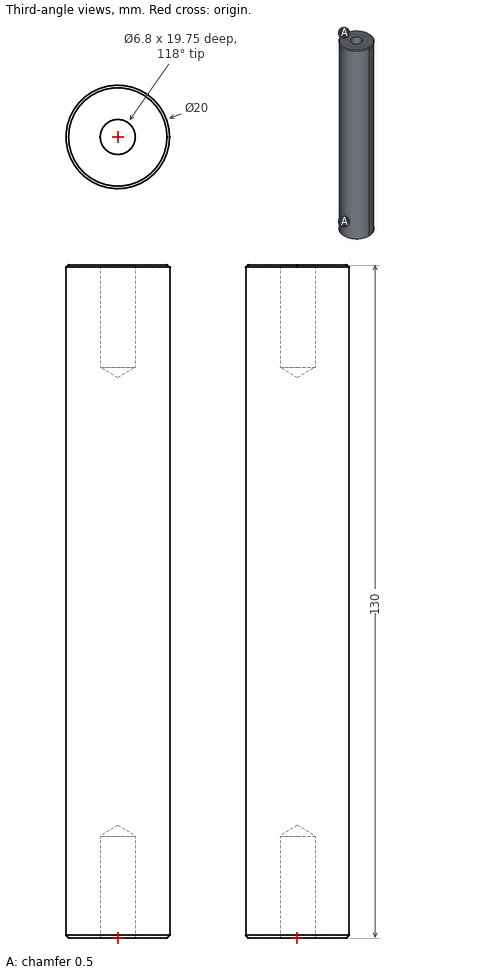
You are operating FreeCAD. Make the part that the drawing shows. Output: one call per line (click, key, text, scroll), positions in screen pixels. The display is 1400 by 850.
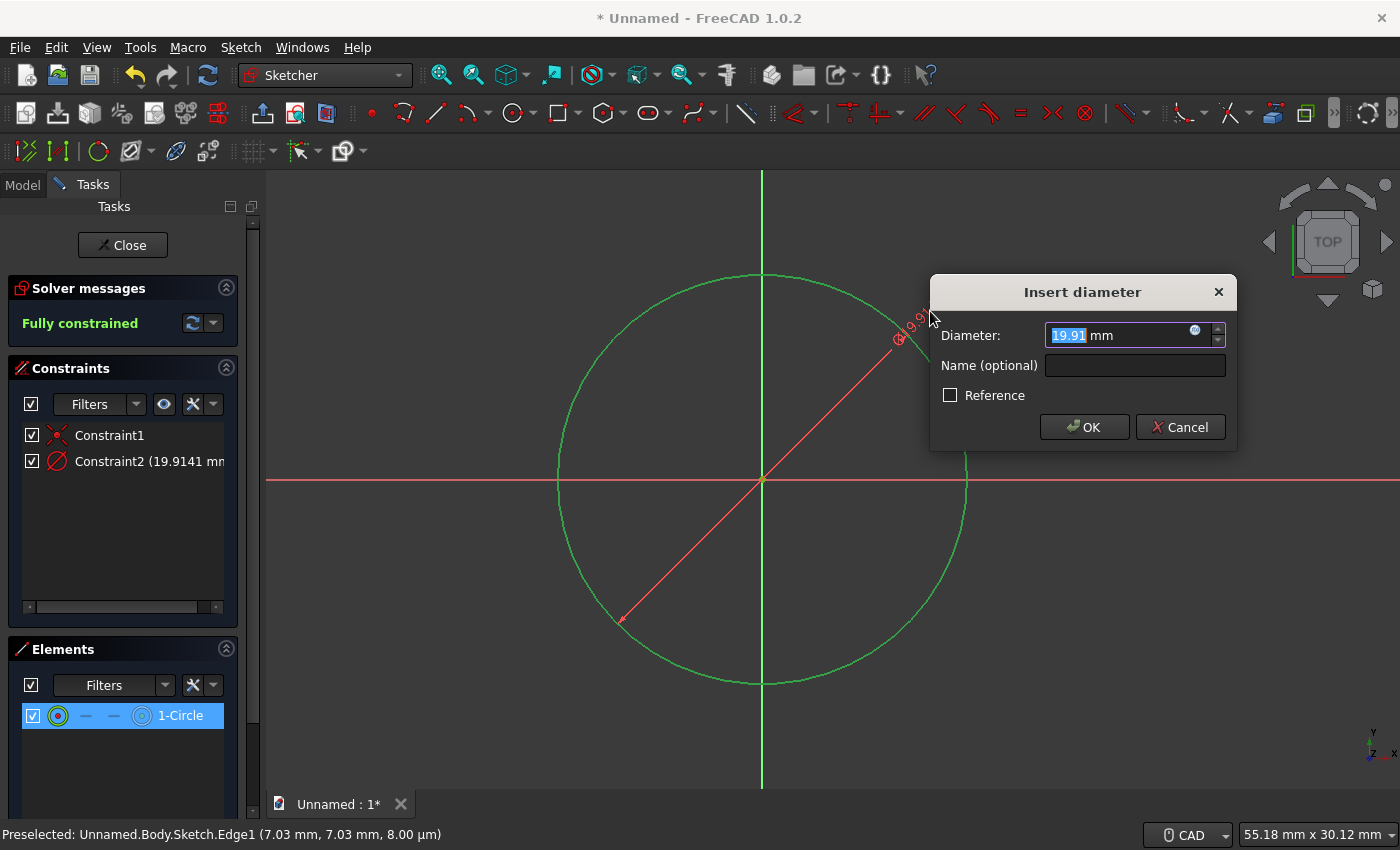
text(20)
key(Return)
key(Escape)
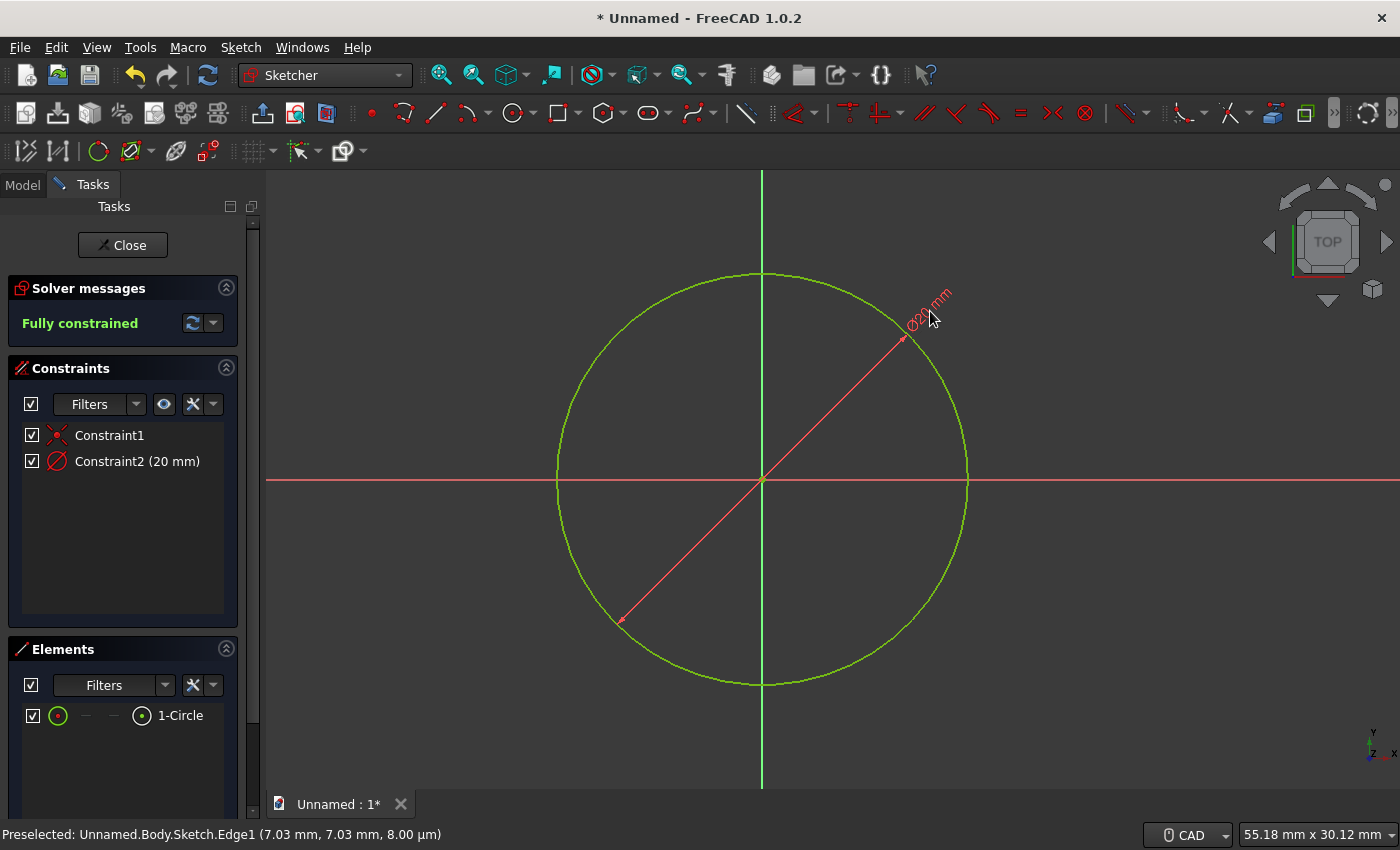
click(123, 245)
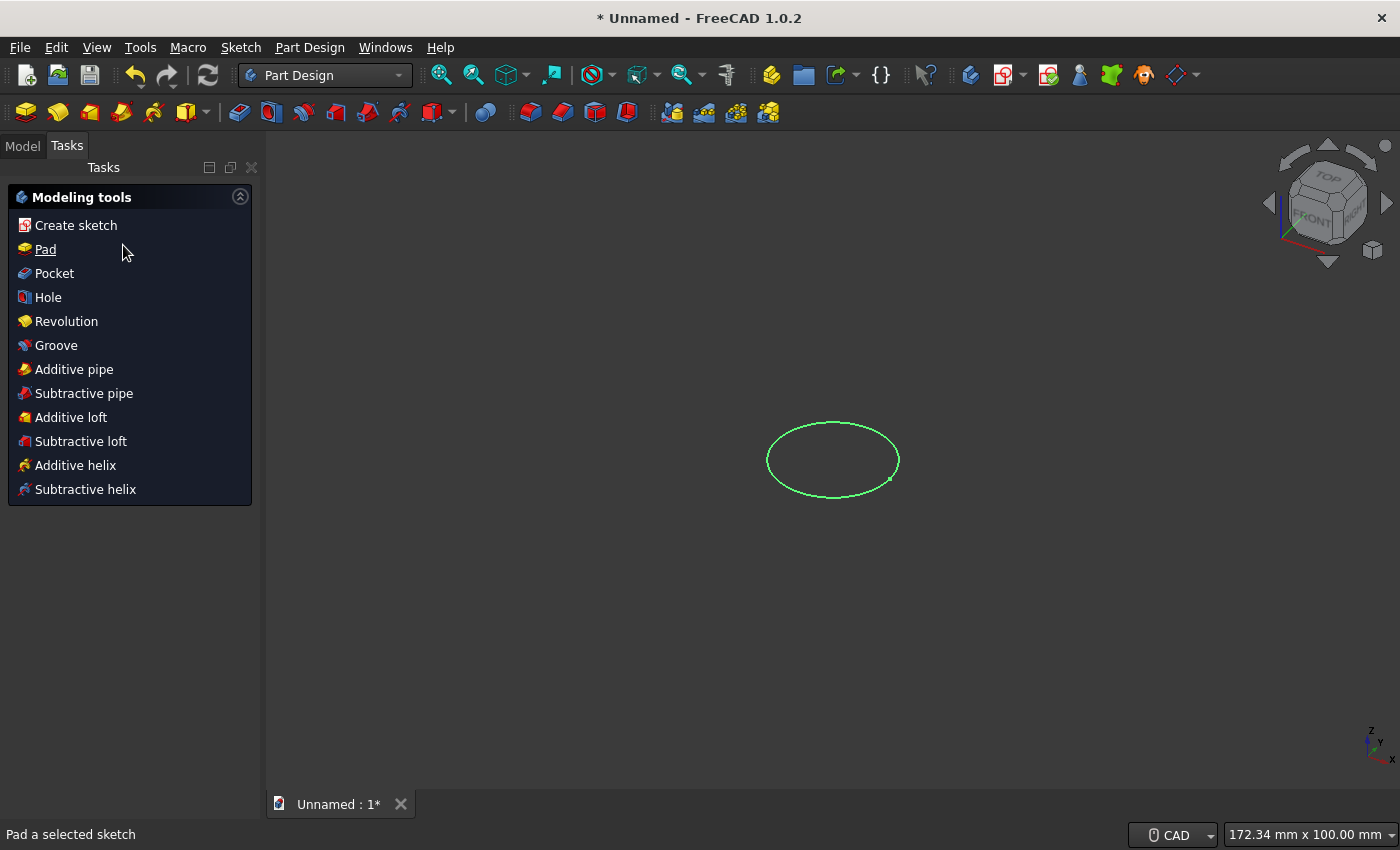
click(26, 112)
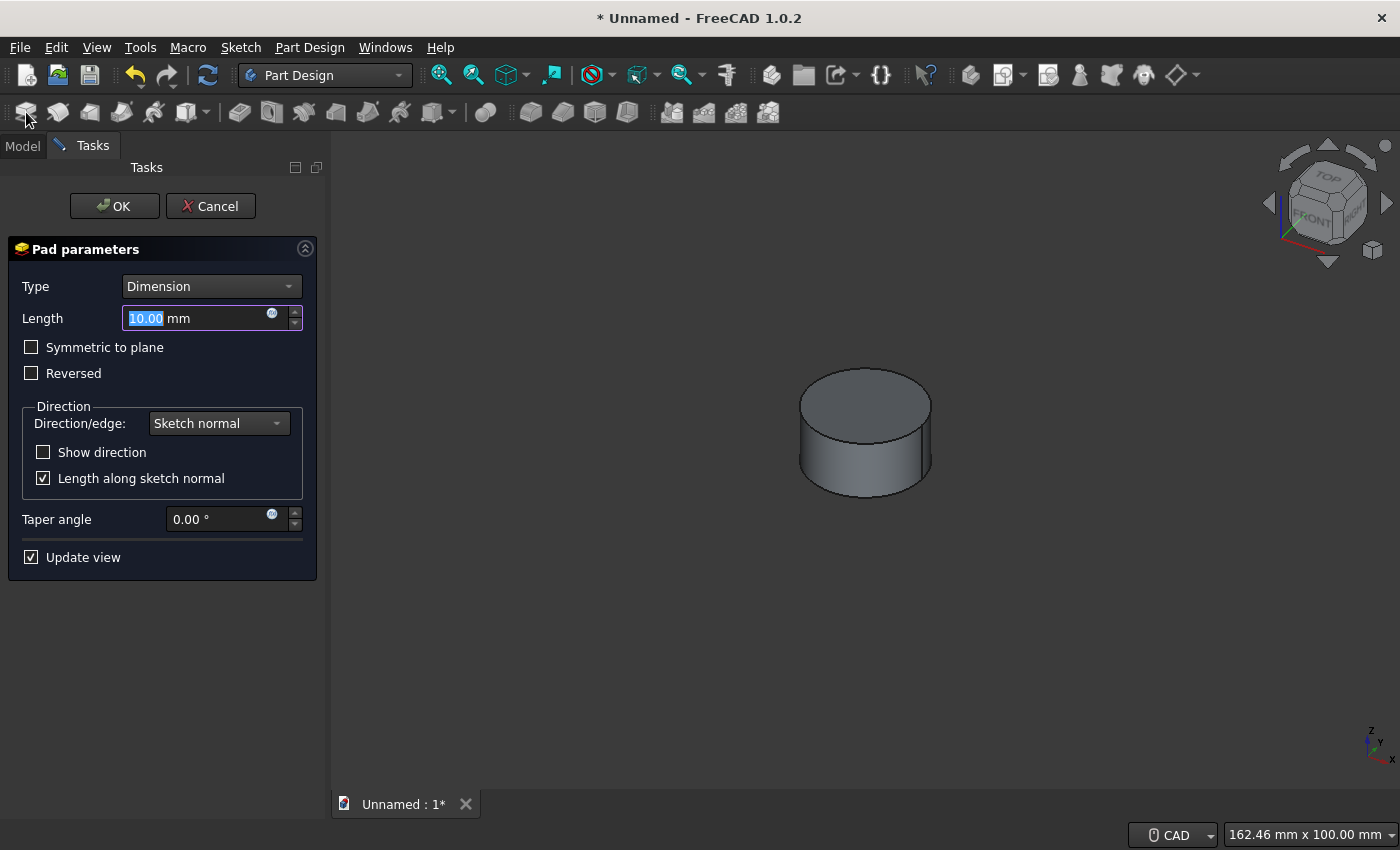
text(130)
key(Tab)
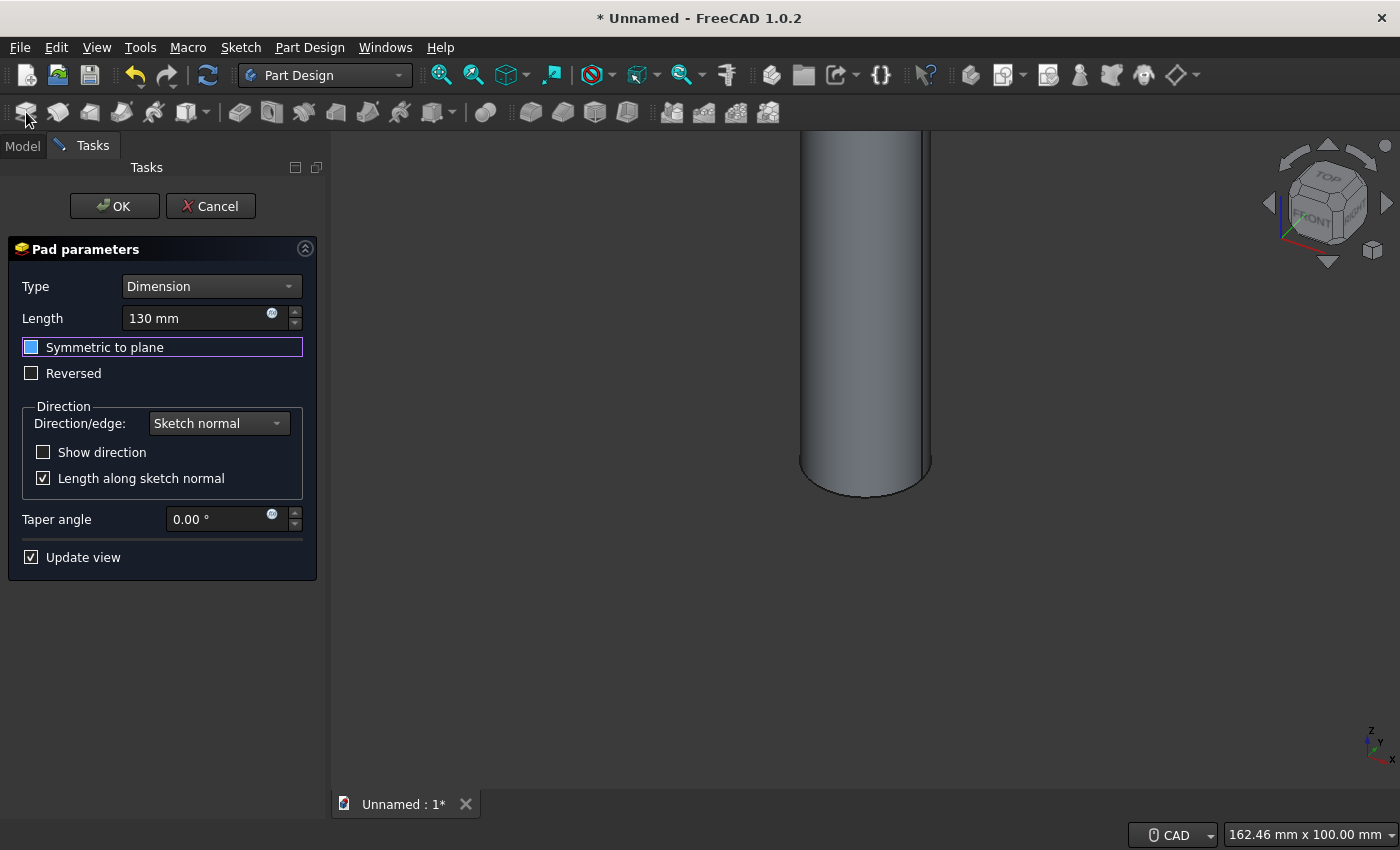
click(115, 206)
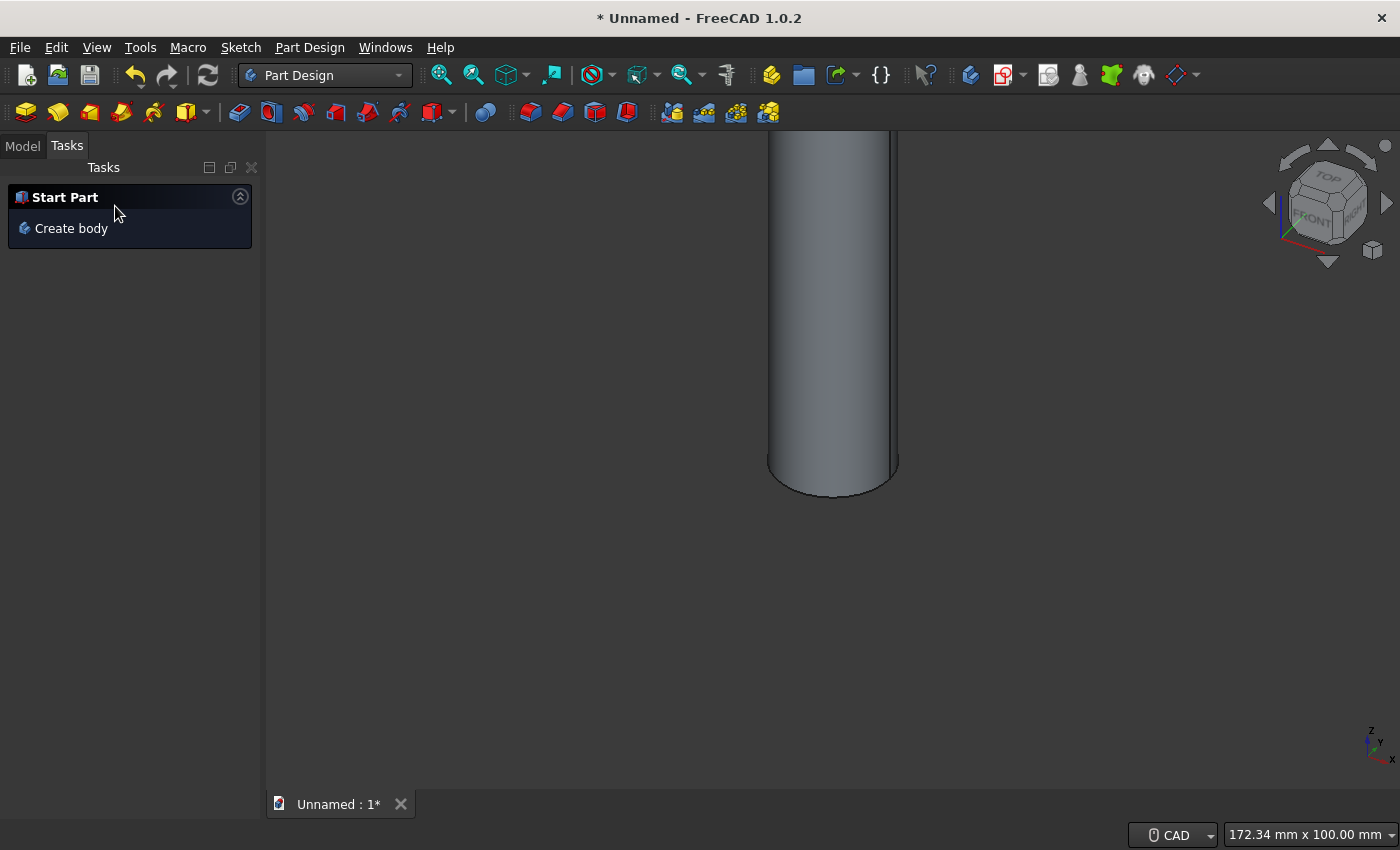
key(v)
key(f)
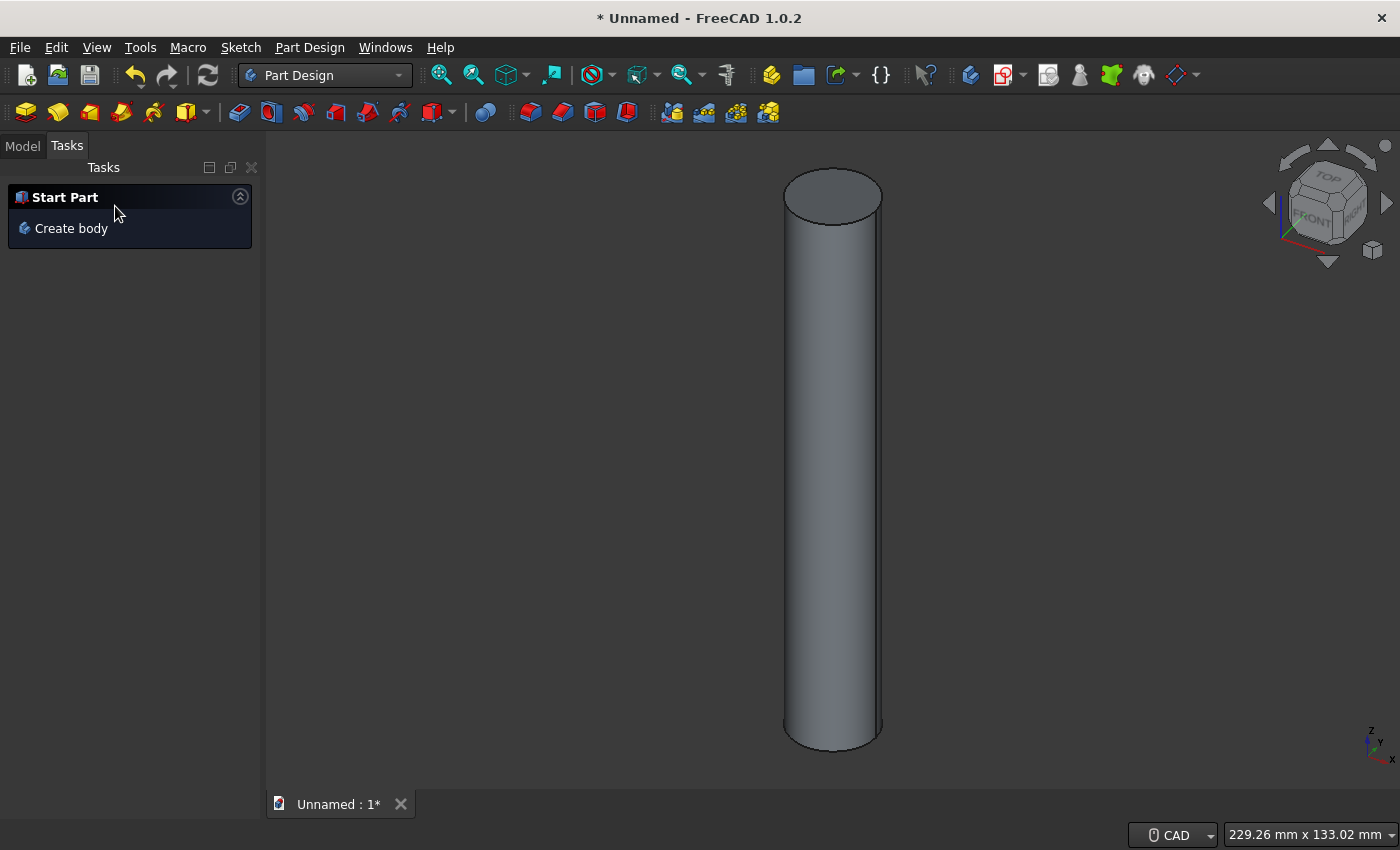
key(5)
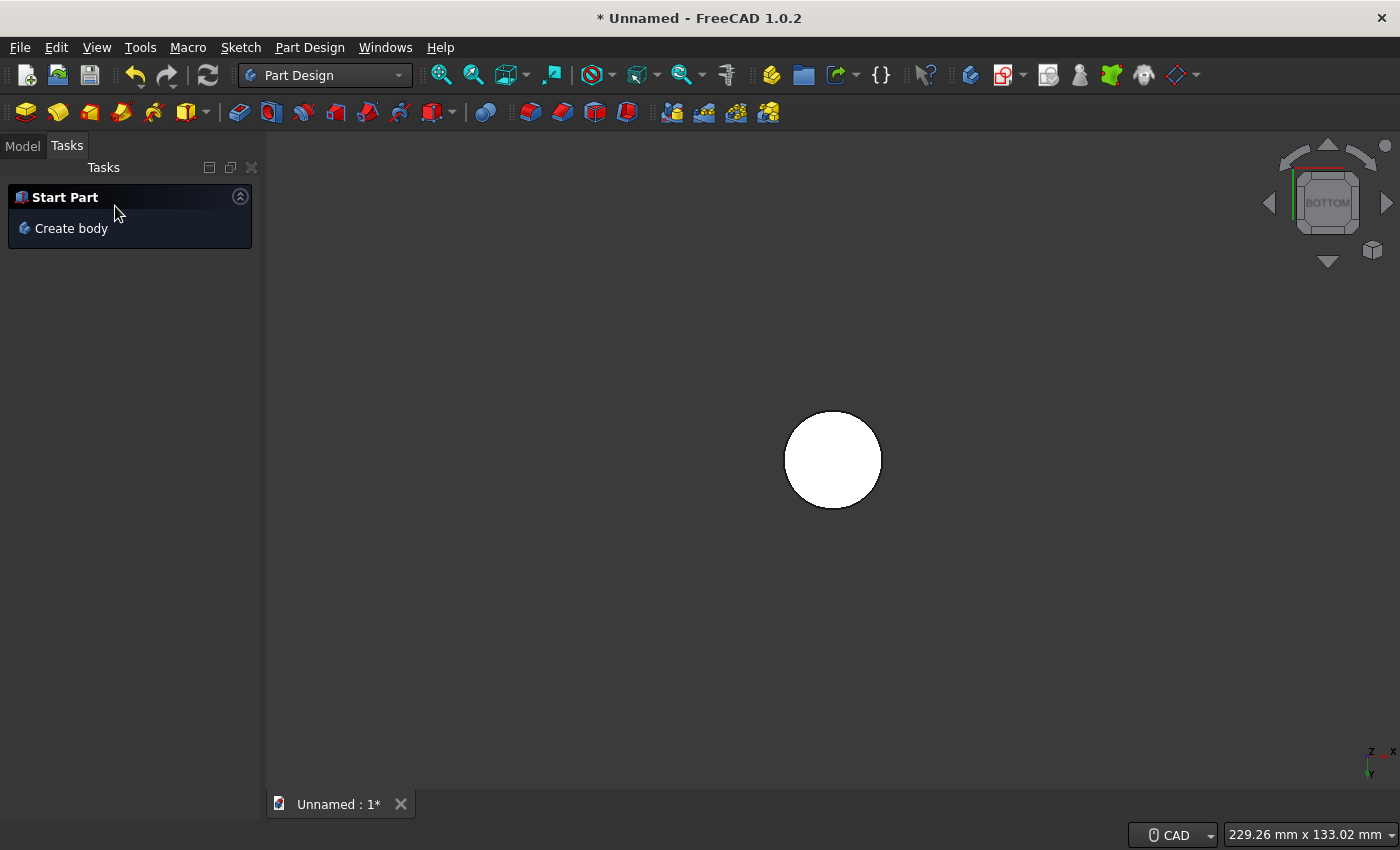
key(v)
key(f)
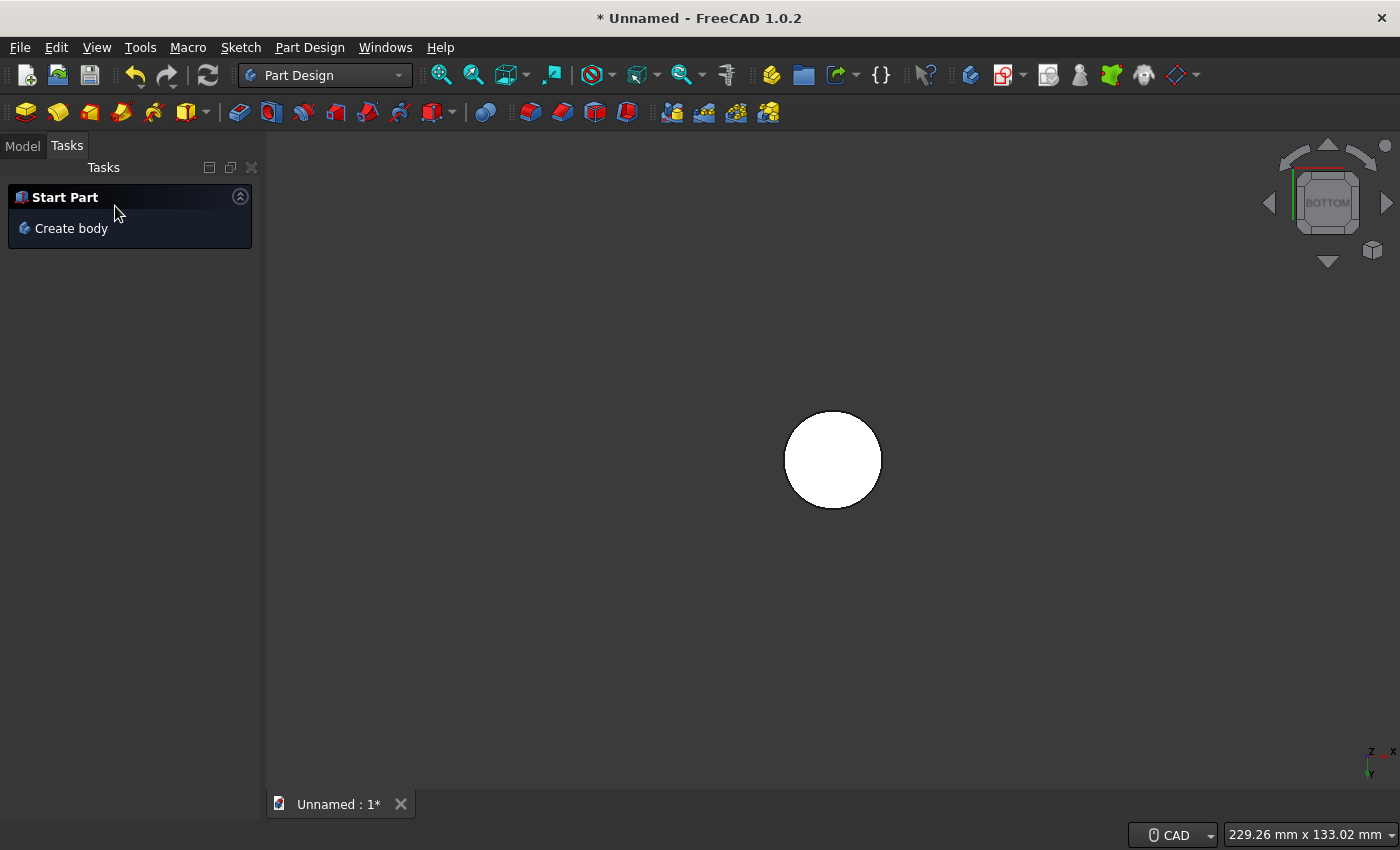
click(833, 459)